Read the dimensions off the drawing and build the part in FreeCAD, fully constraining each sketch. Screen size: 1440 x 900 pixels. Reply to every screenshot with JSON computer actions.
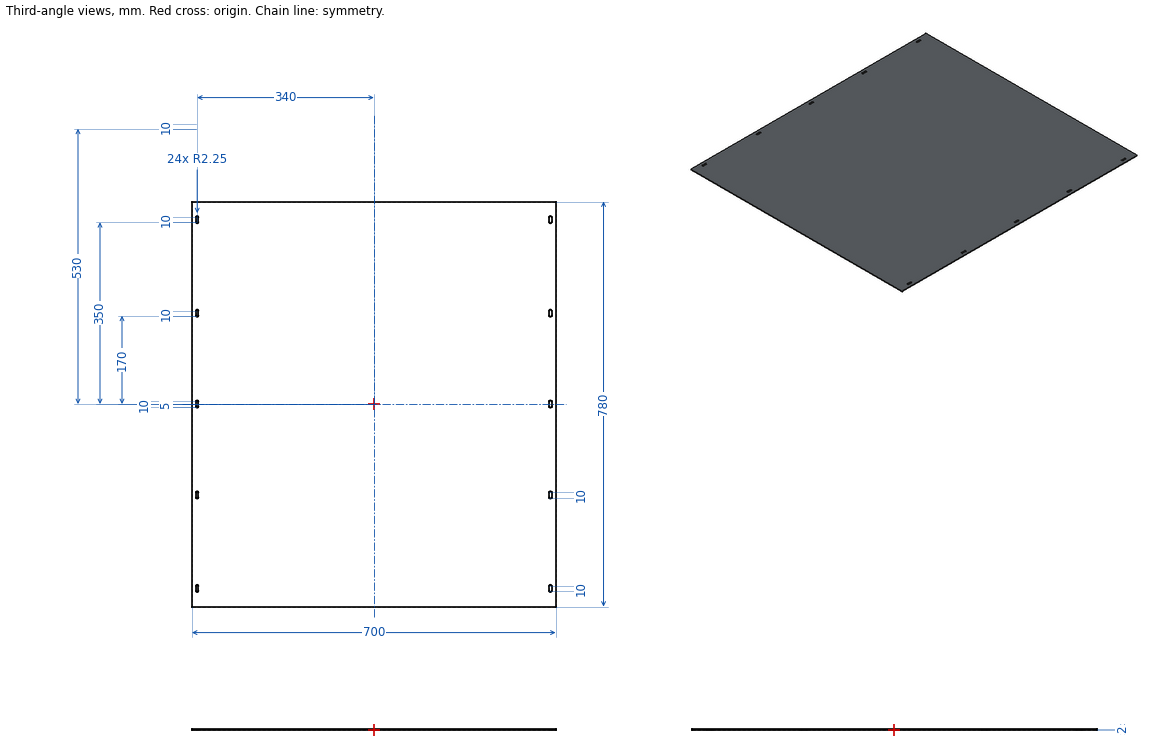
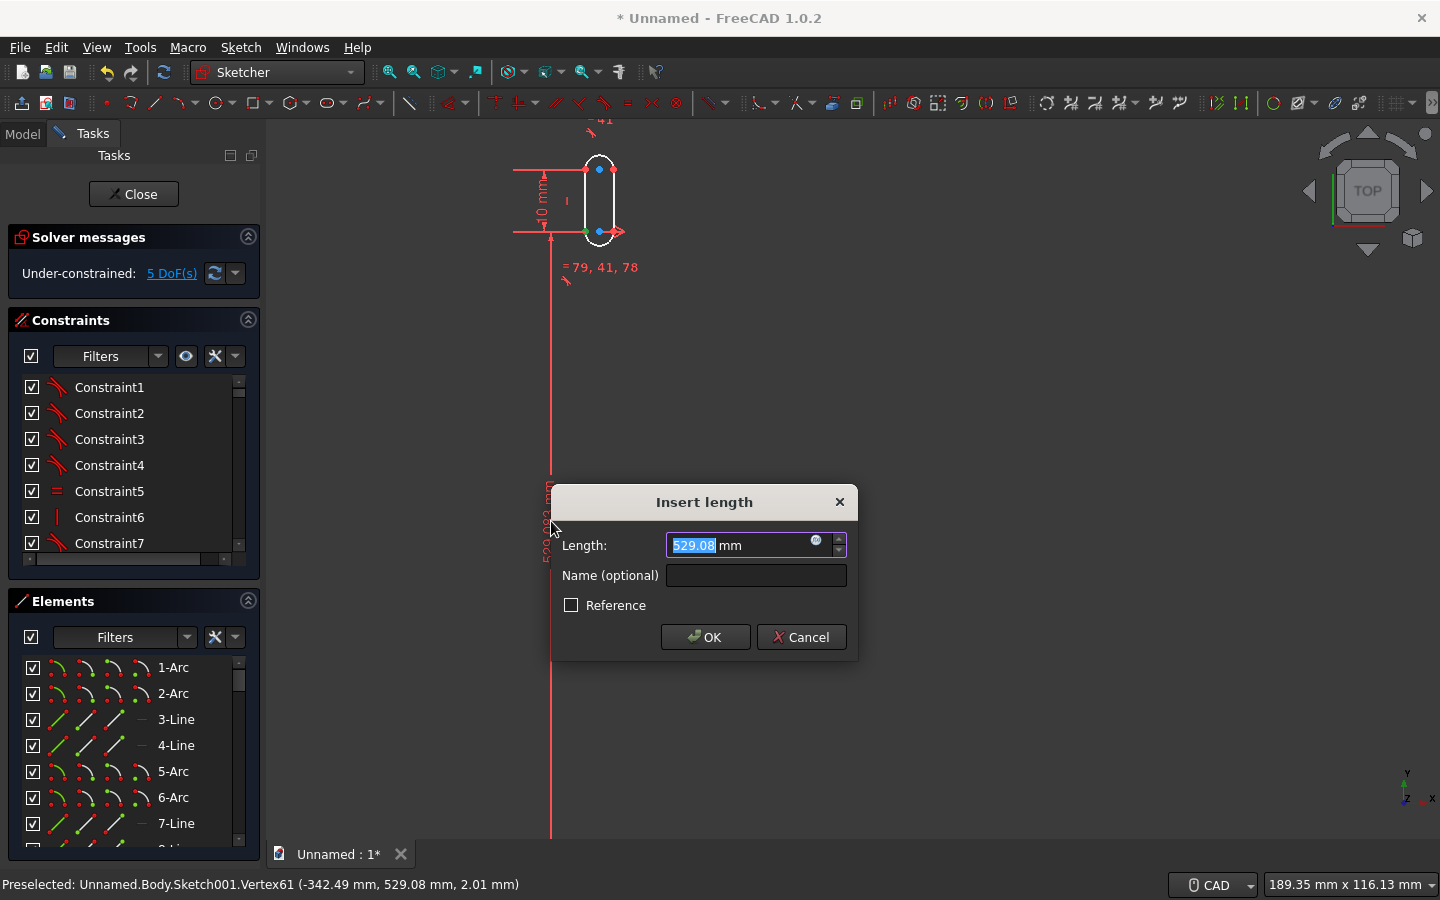
{"action": "type", "text": "530"}
{"action": "key", "text": "Return"}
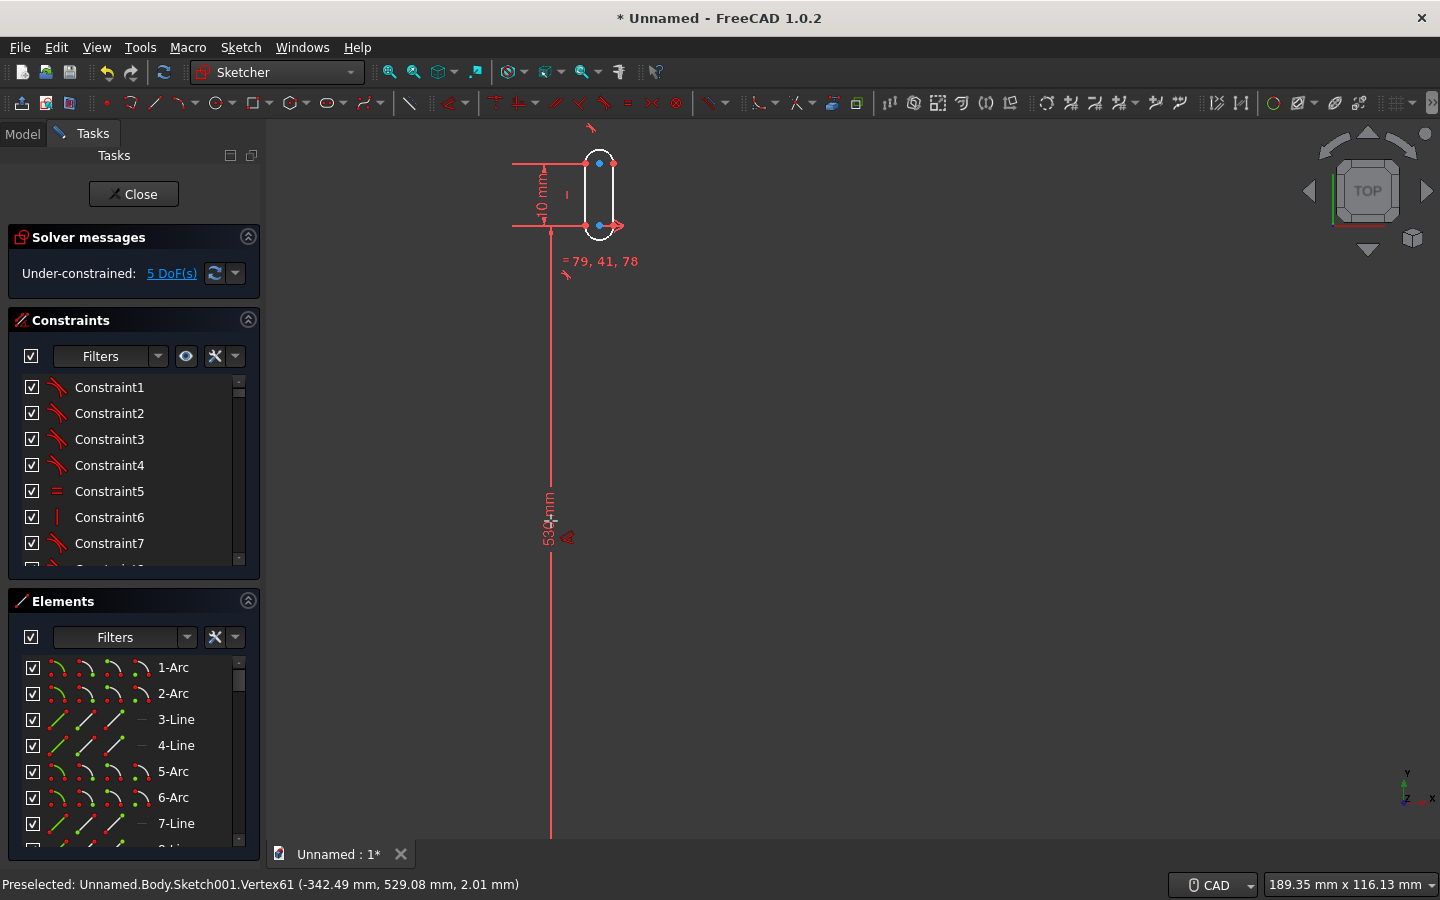
{"action": "scroll", "coordinate": [593, 232], "scroll_direction": "down", "scroll_amount": 12}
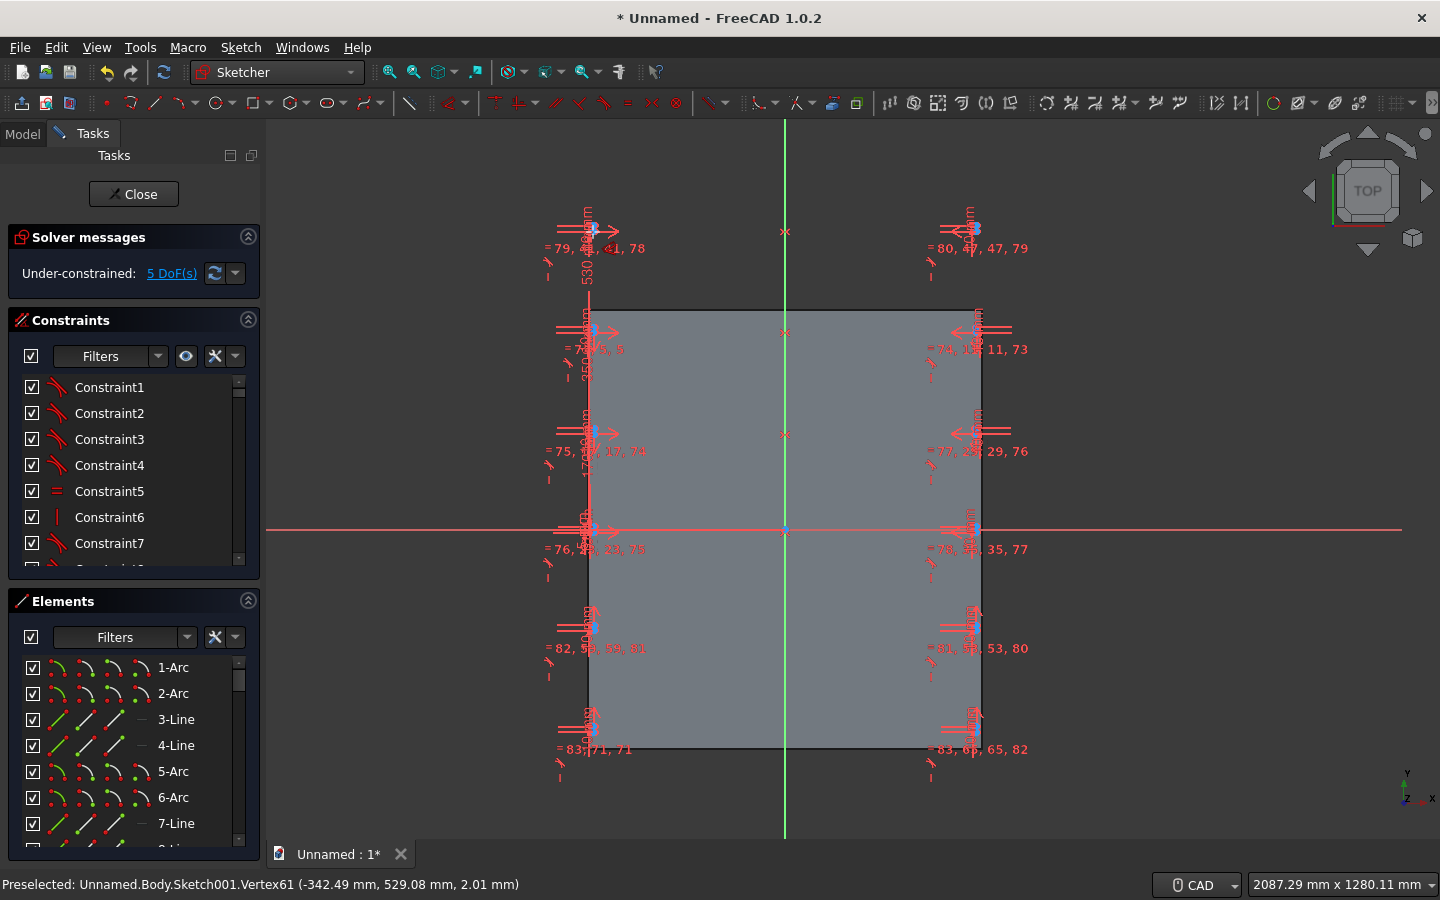
{"action": "scroll", "coordinate": [594, 333], "scroll_direction": "up", "scroll_amount": 12}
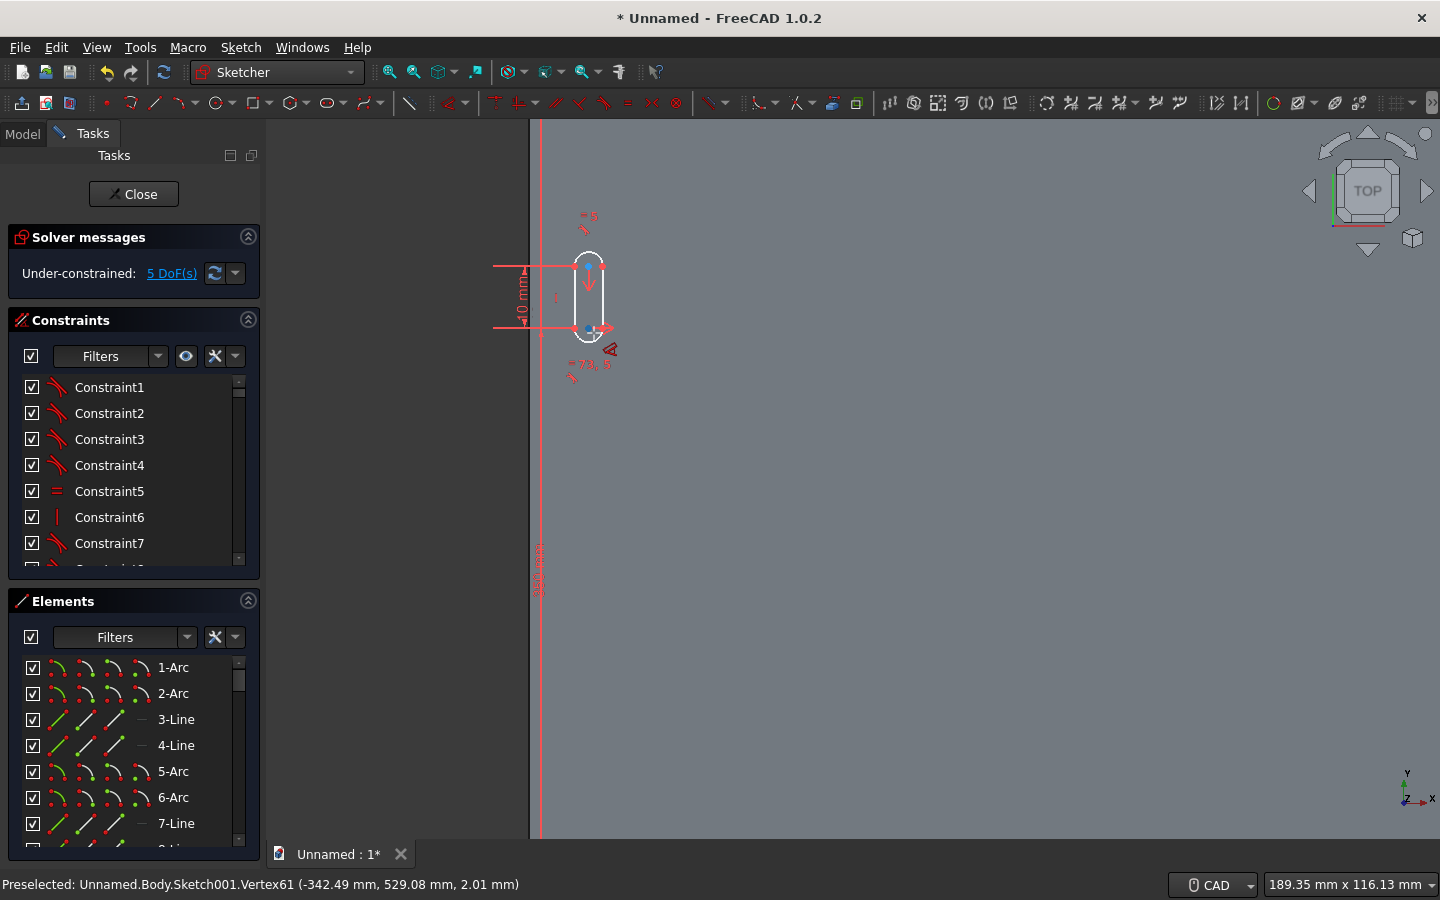
{"action": "left_click", "coordinate": [589, 328]}
{"action": "left_click", "coordinate": [932, 294]}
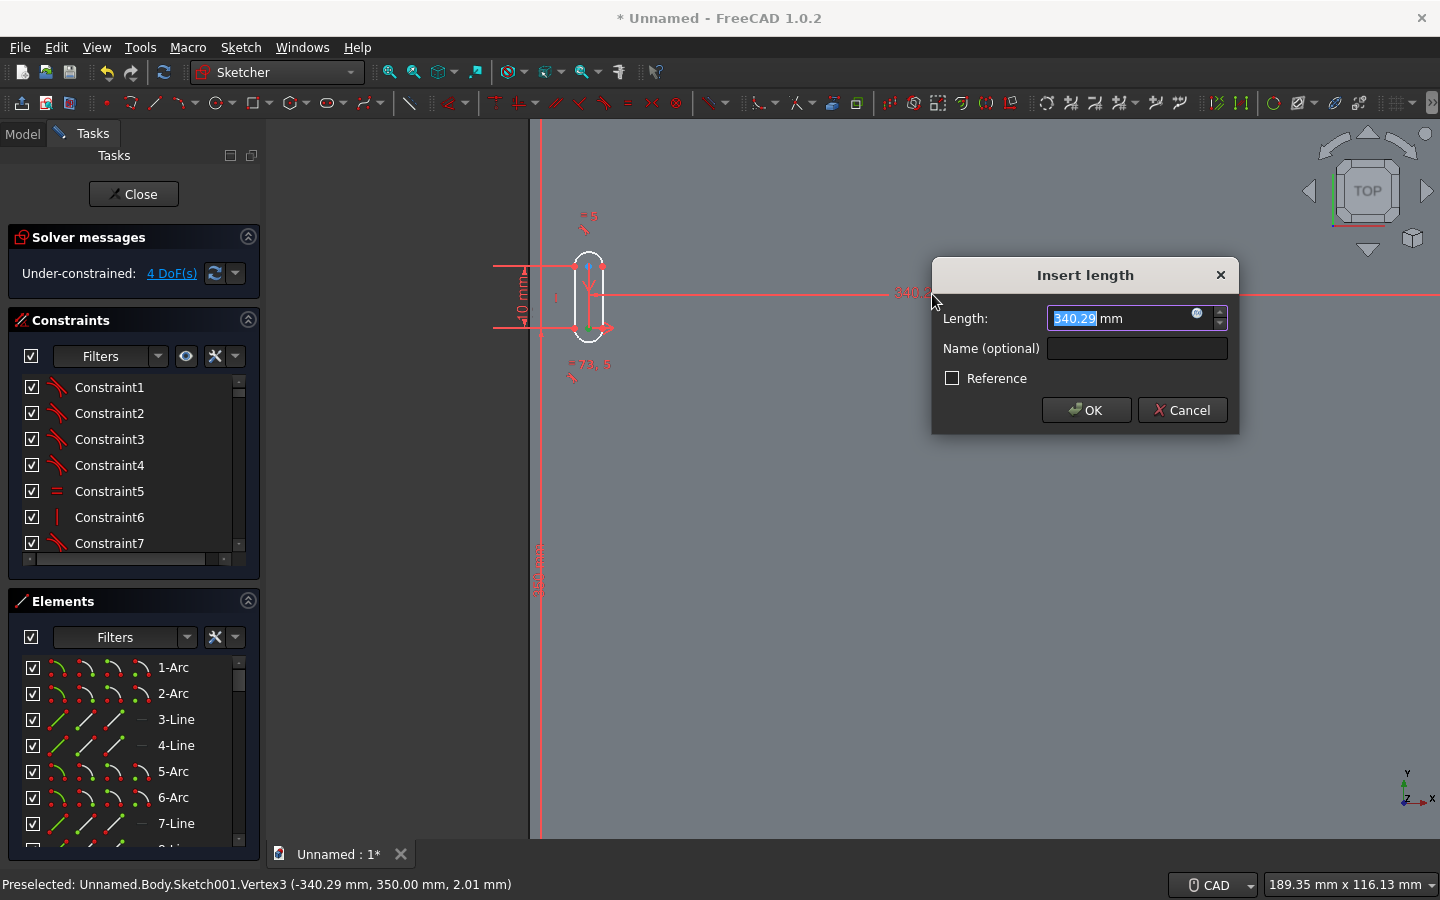
{"action": "type", "text": "340"}
{"action": "key", "text": "Return"}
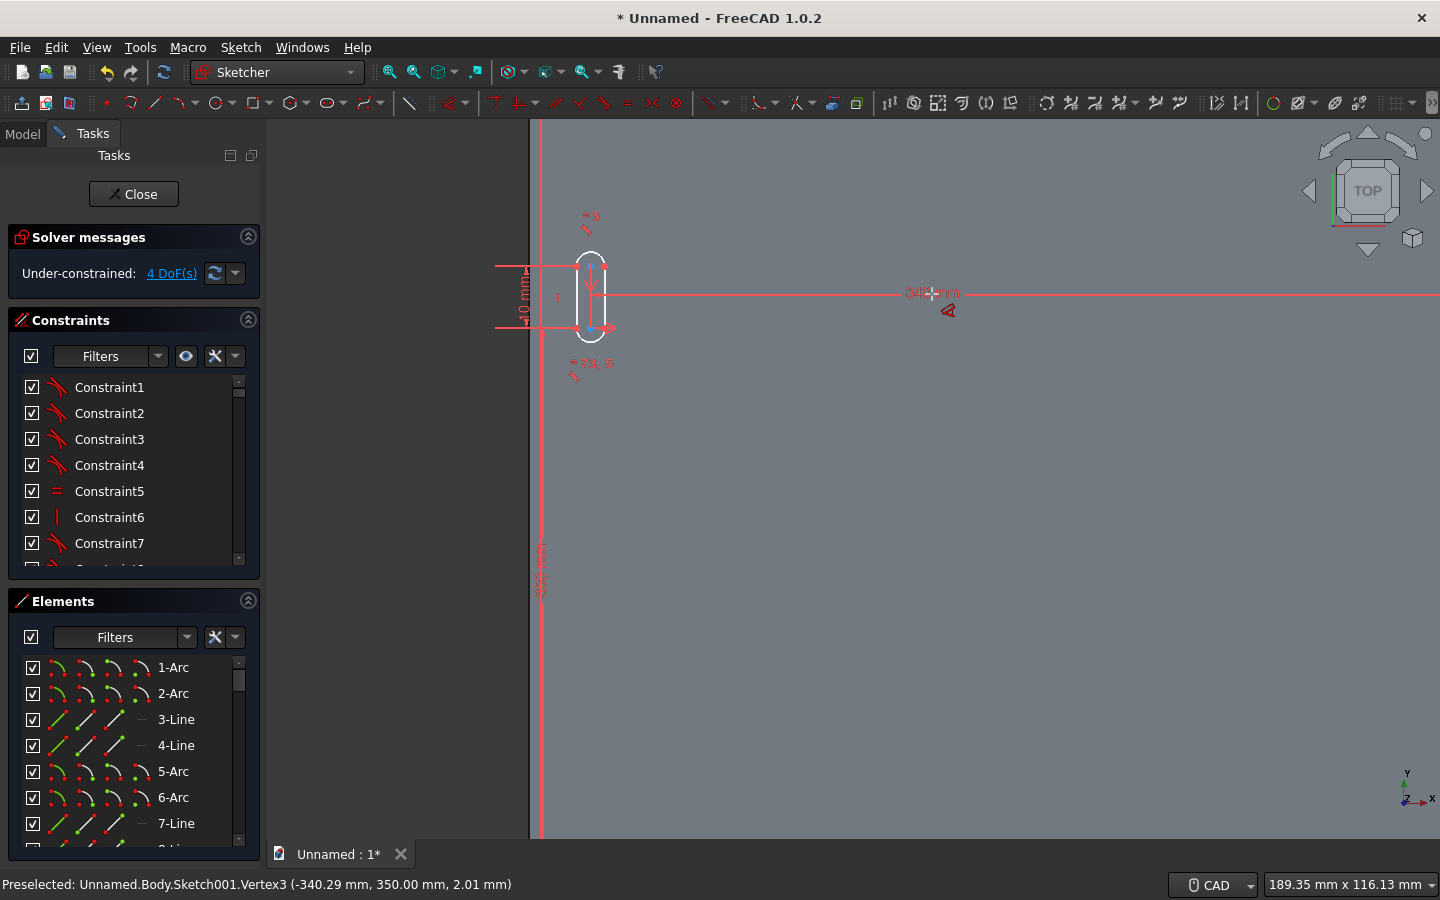
{"action": "scroll", "coordinate": [594, 333], "scroll_direction": "down", "scroll_amount": 12}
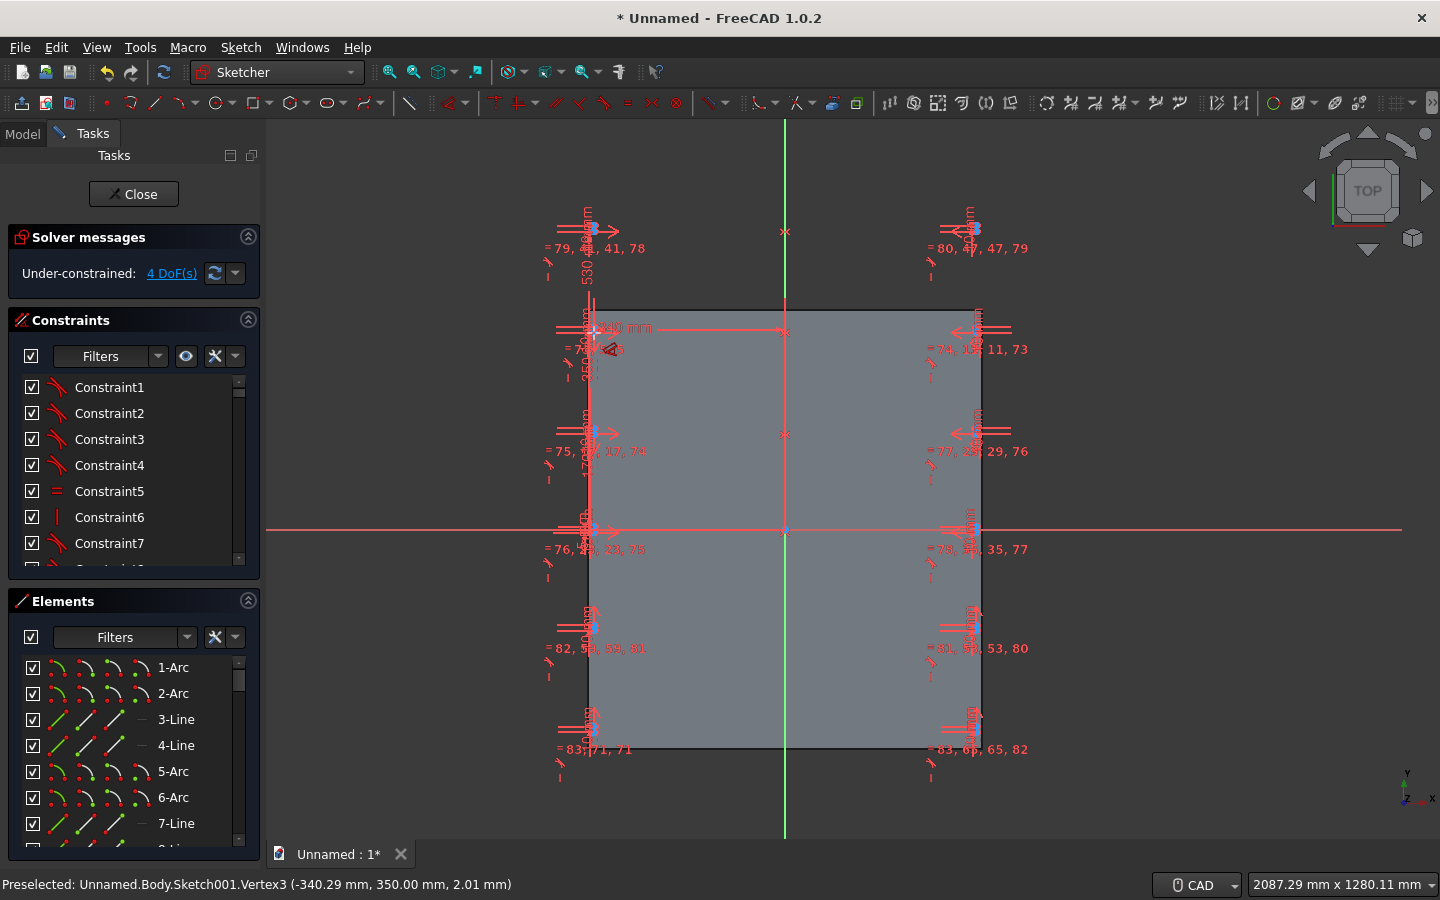
{"action": "scroll", "coordinate": [594, 434], "scroll_direction": "up", "scroll_amount": 12}